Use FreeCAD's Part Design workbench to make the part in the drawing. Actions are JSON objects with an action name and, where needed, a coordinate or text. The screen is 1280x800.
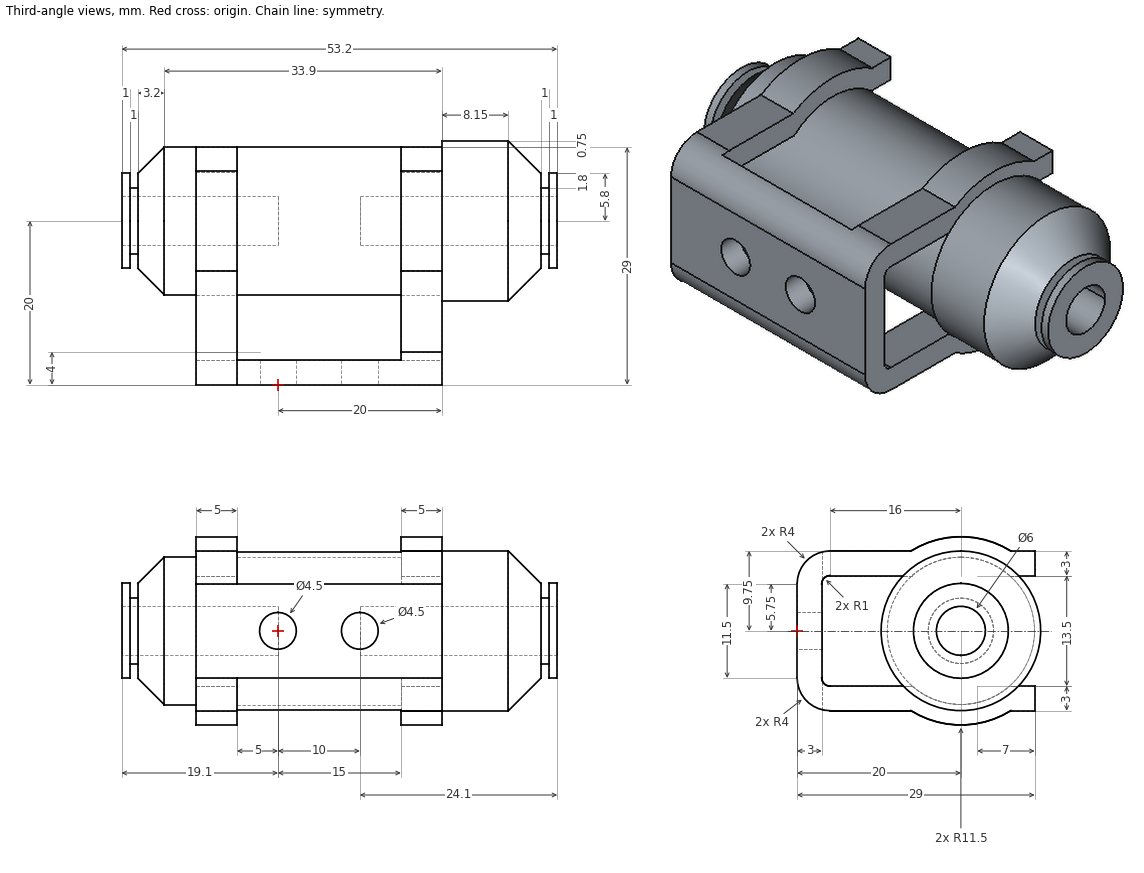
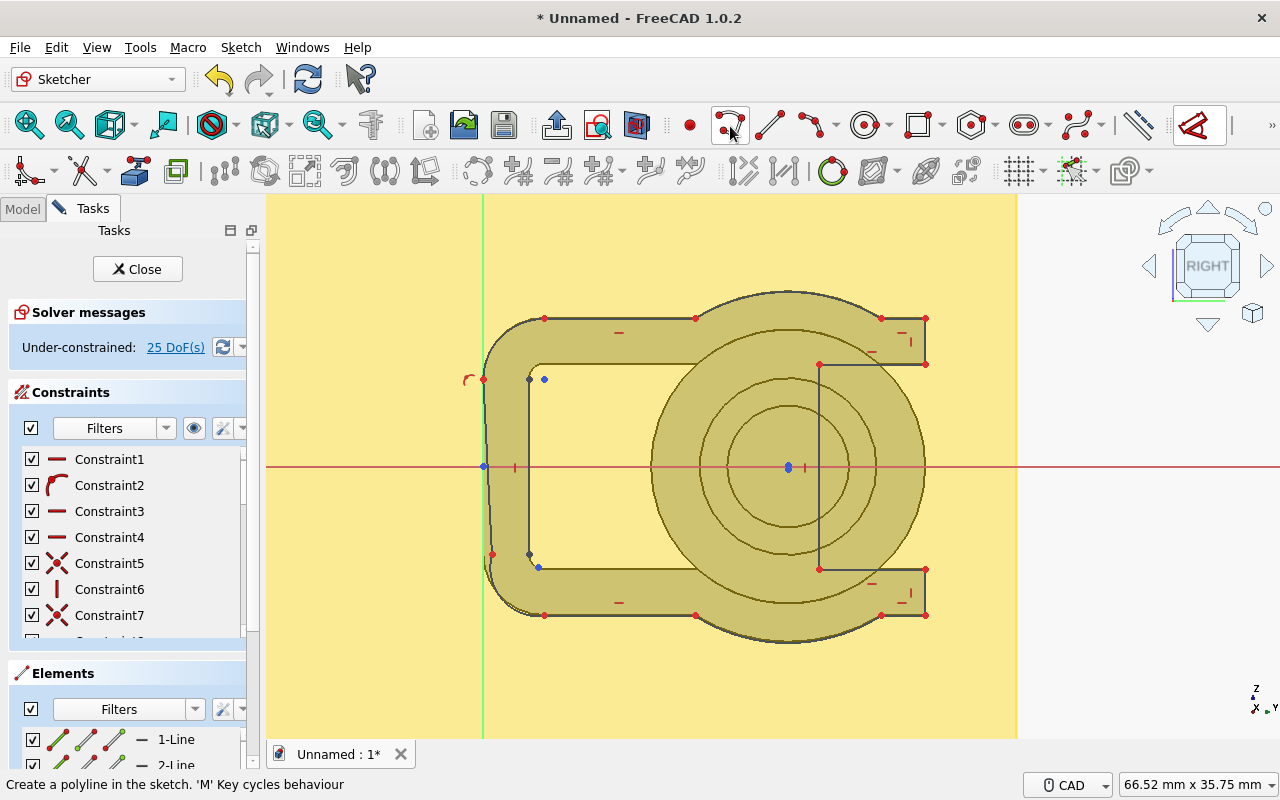
{"action": "left_click", "coordinate": [544, 364]}
{"action": "left_click", "coordinate": [788, 364]}
{"action": "left_click", "coordinate": [788, 569]}
{"action": "left_click", "coordinate": [544, 569]}
{"action": "right_click", "coordinate": [544, 569]}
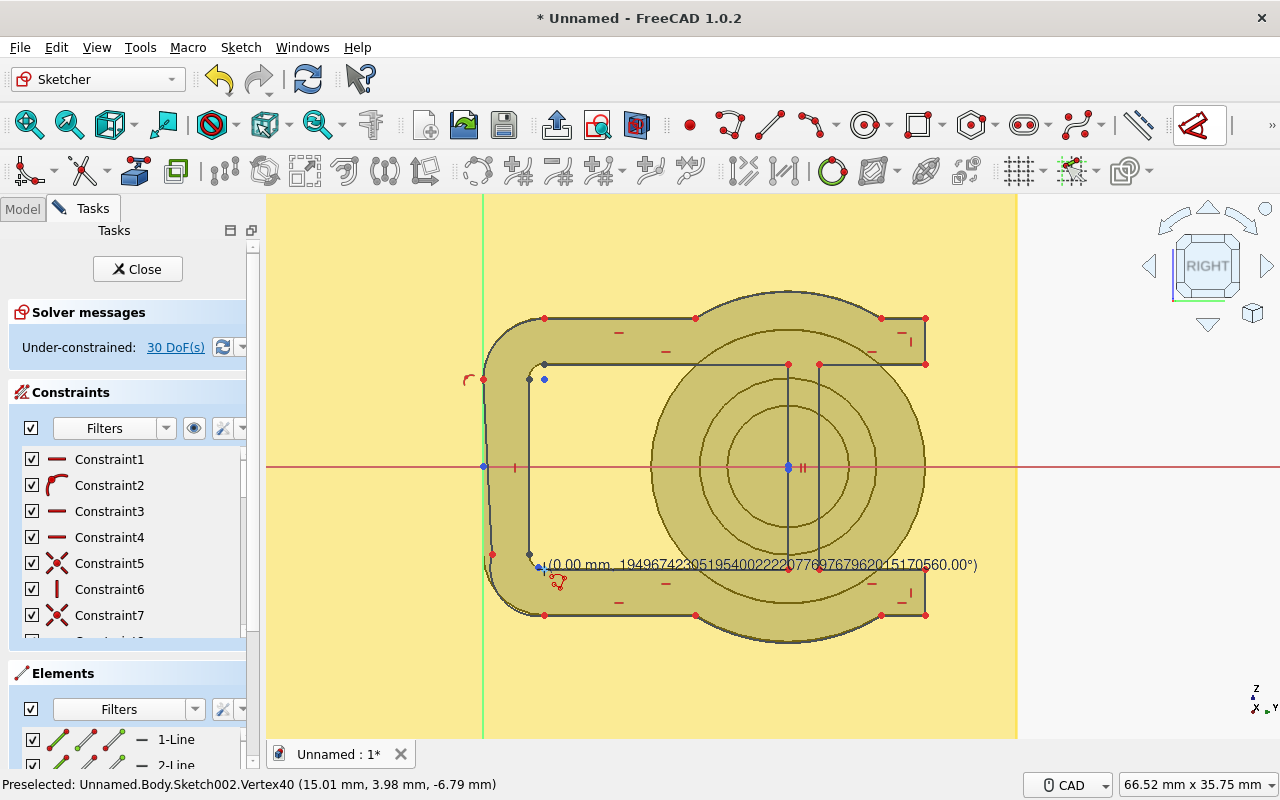
{"action": "left_click", "coordinate": [812, 126]}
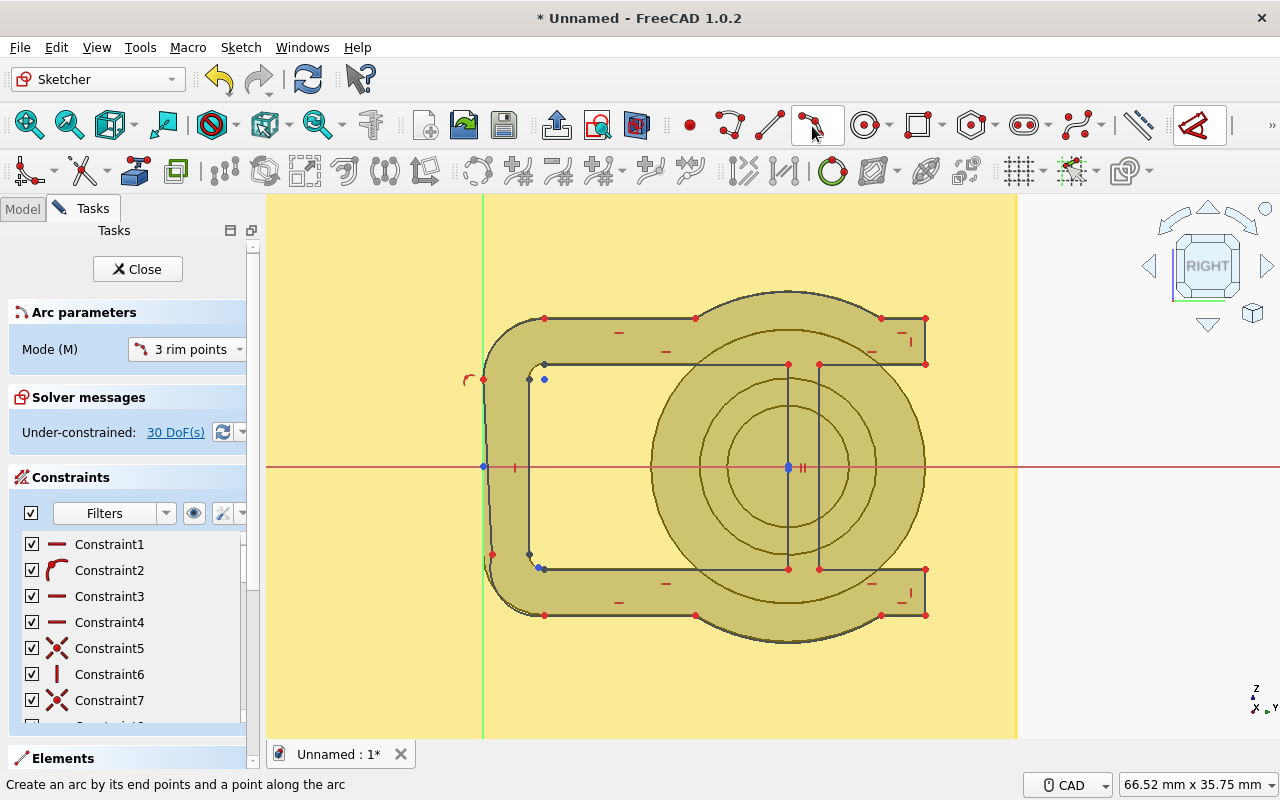
{"action": "left_click", "coordinate": [529, 380]}
{"action": "left_click", "coordinate": [544, 365]}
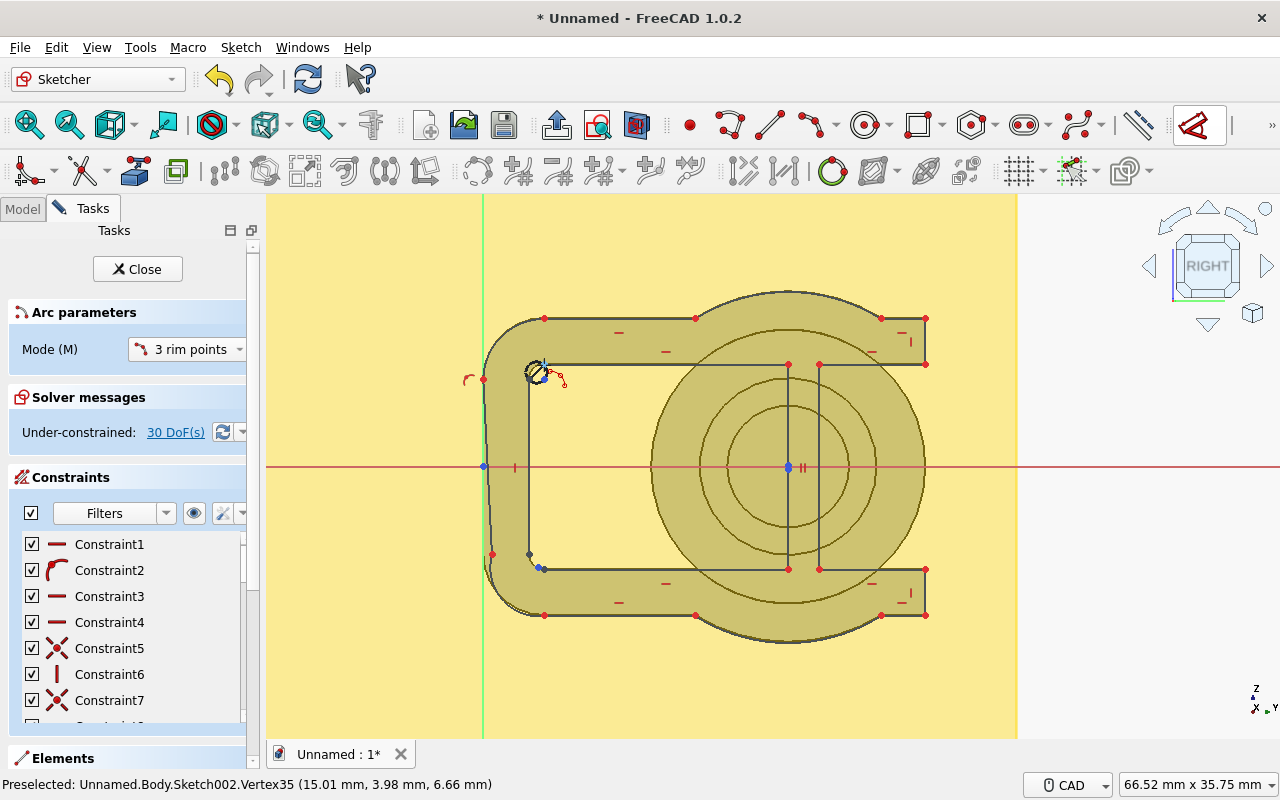
{"action": "scroll", "coordinate": [533, 368], "scroll_direction": "up", "scroll_amount": 7}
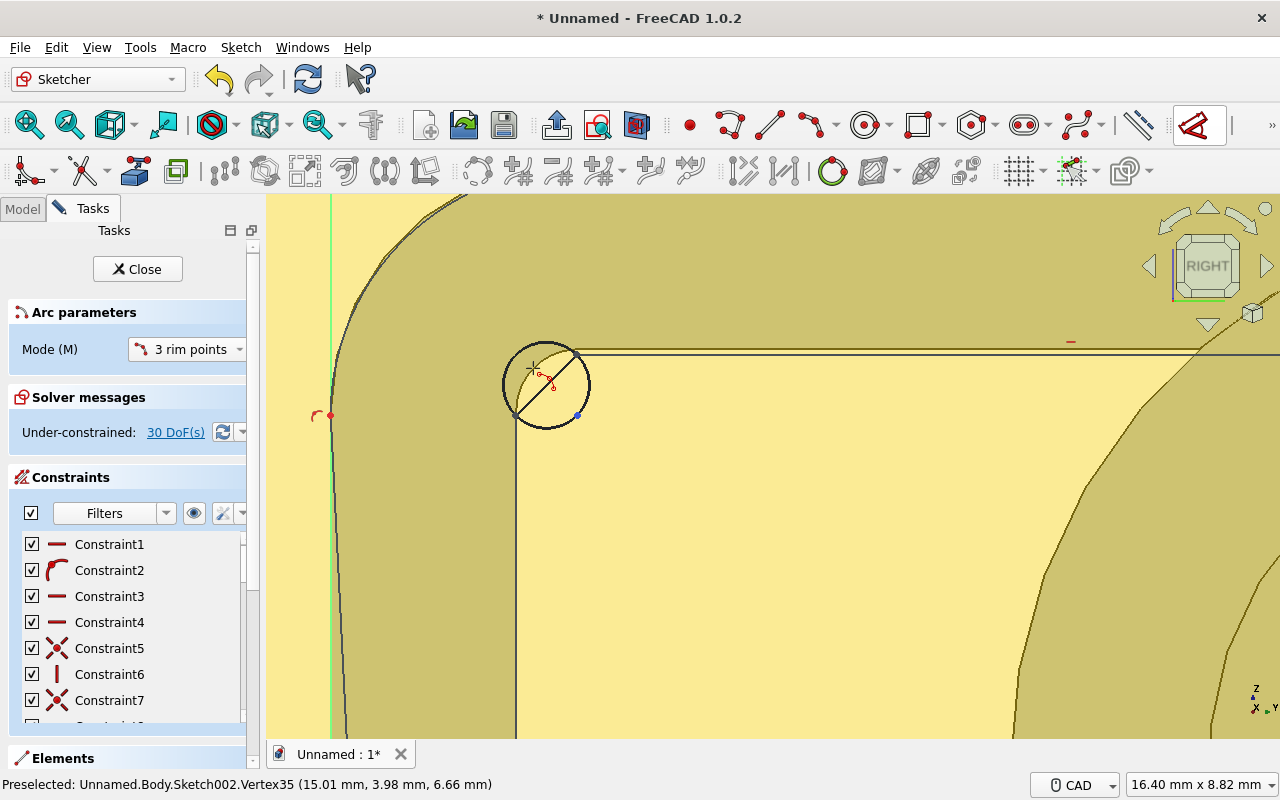
{"action": "left_click", "coordinate": [534, 367]}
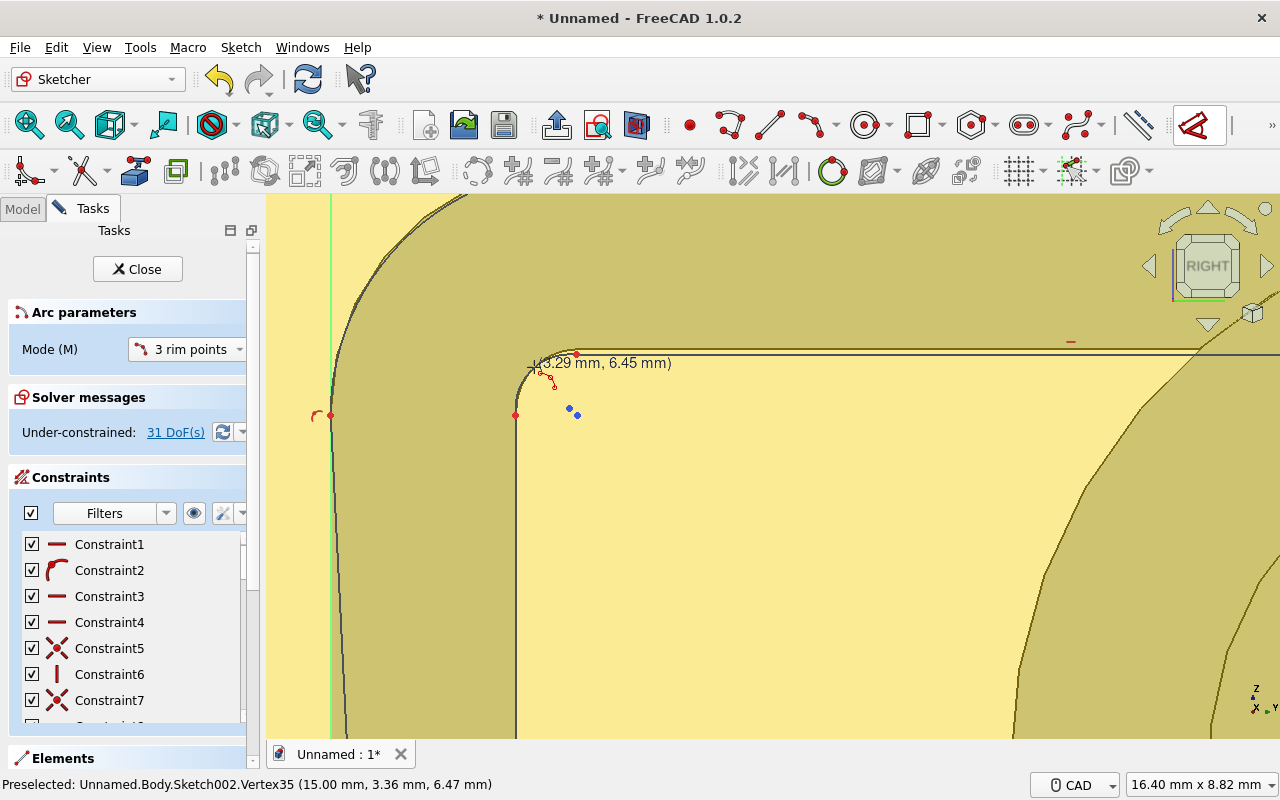
{"action": "scroll", "coordinate": [533, 368], "scroll_direction": "down", "scroll_amount": 7}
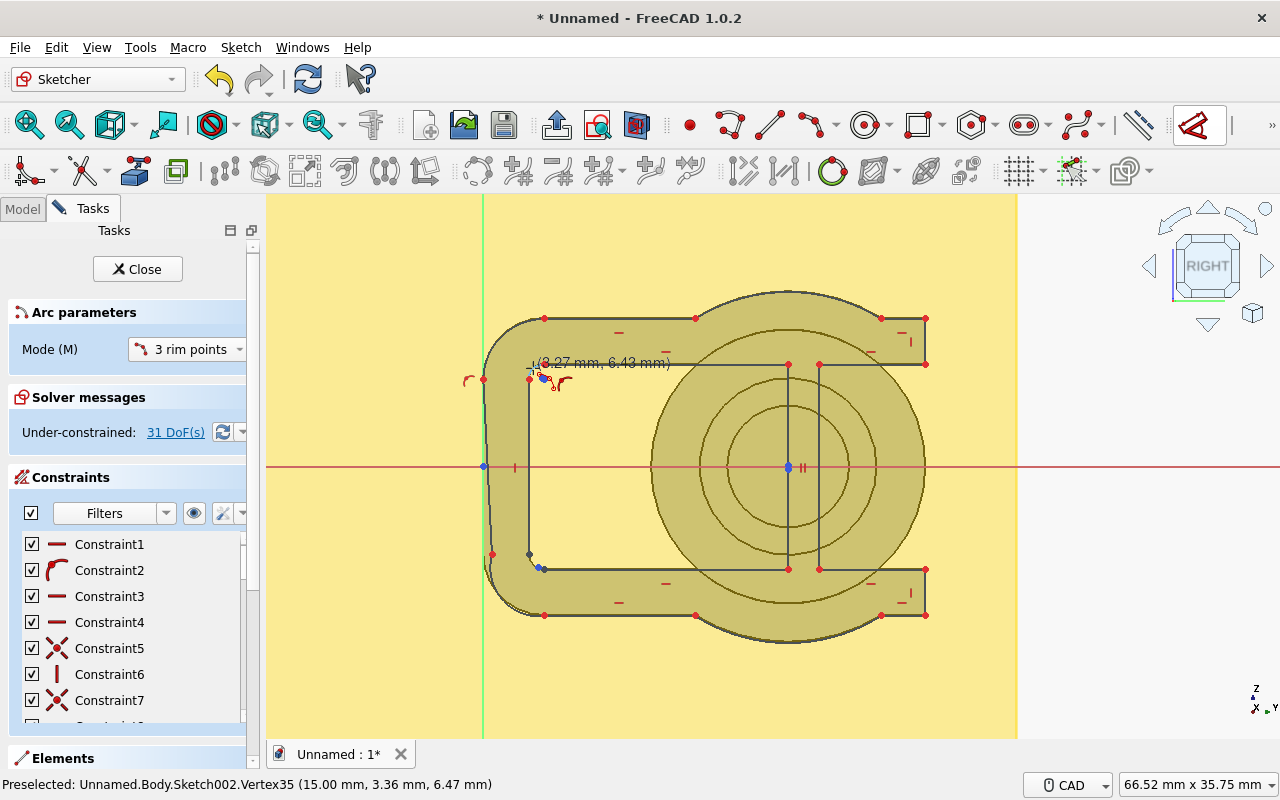
{"action": "left_click", "coordinate": [544, 570]}
{"action": "left_click", "coordinate": [529, 555]}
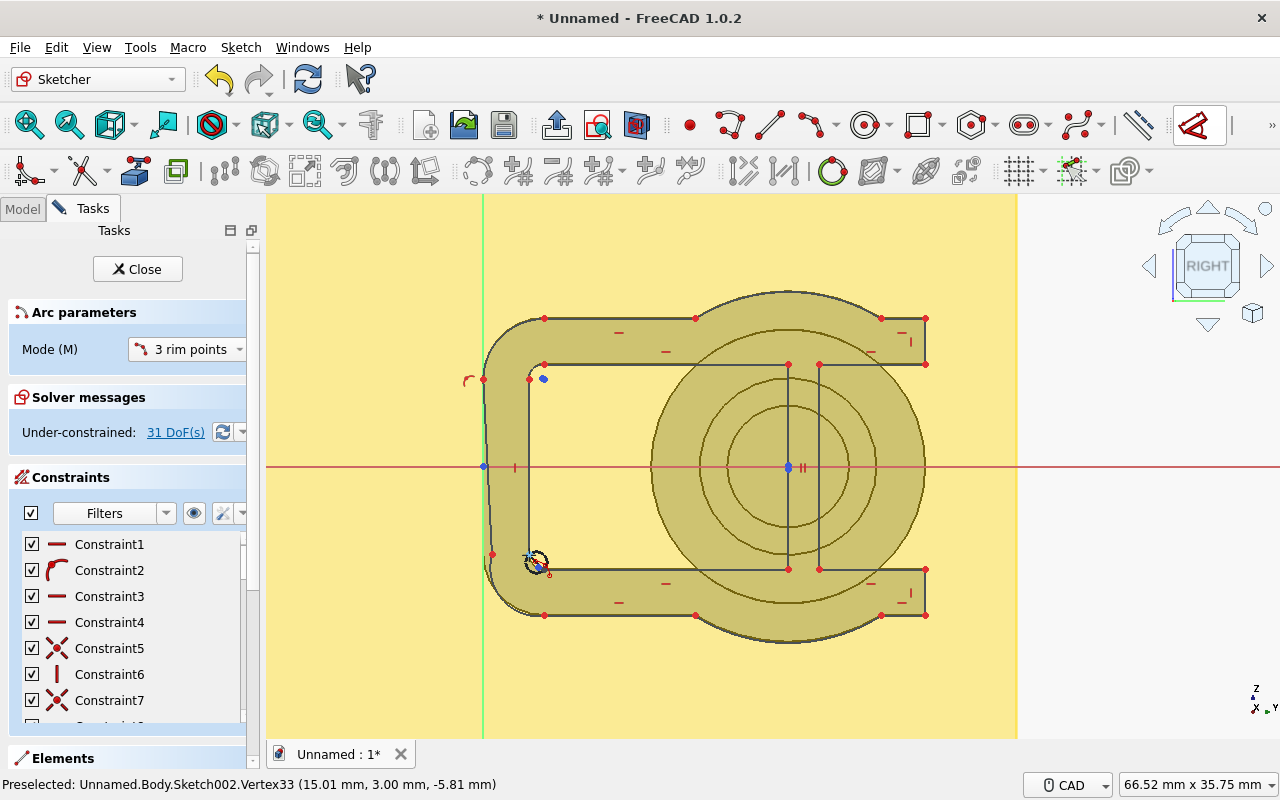
{"action": "scroll", "coordinate": [534, 565], "scroll_direction": "up", "scroll_amount": 7}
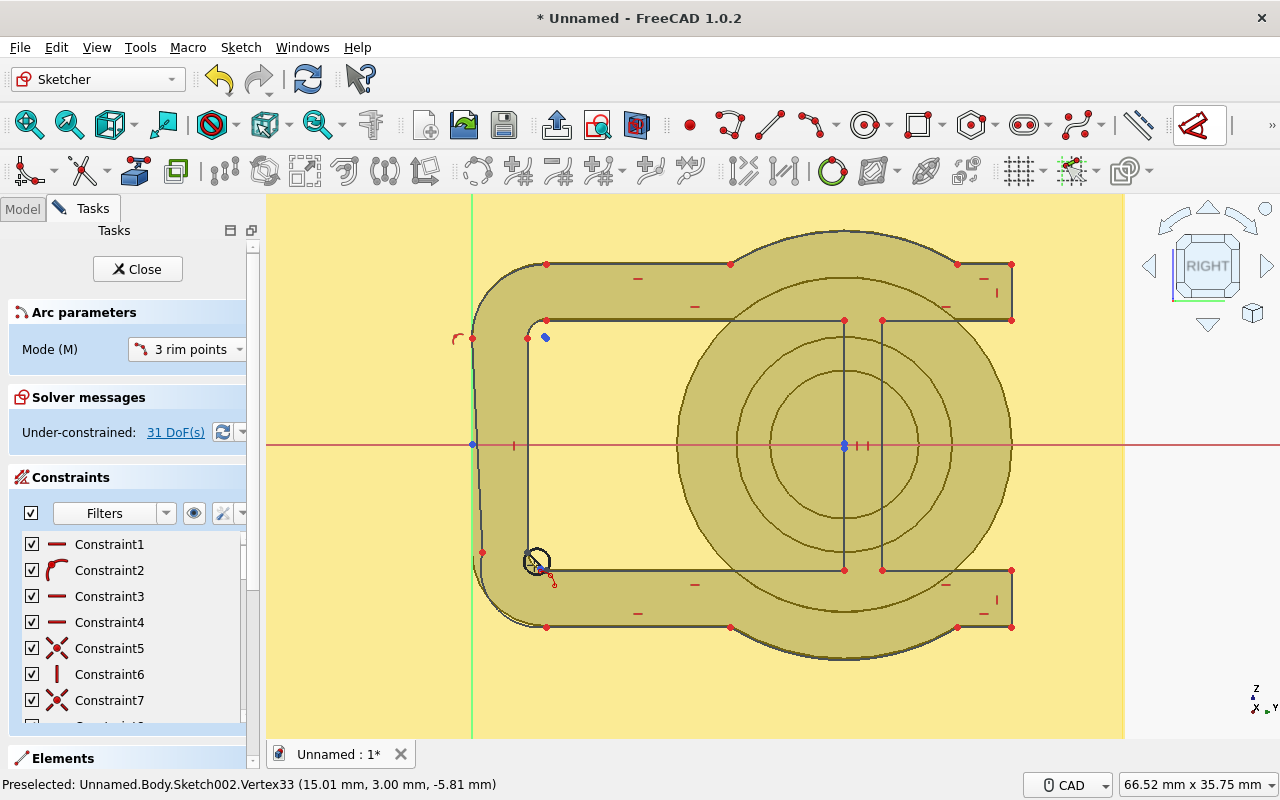
{"action": "left_click", "coordinate": [531, 563]}
{"action": "key", "text": "Escape"}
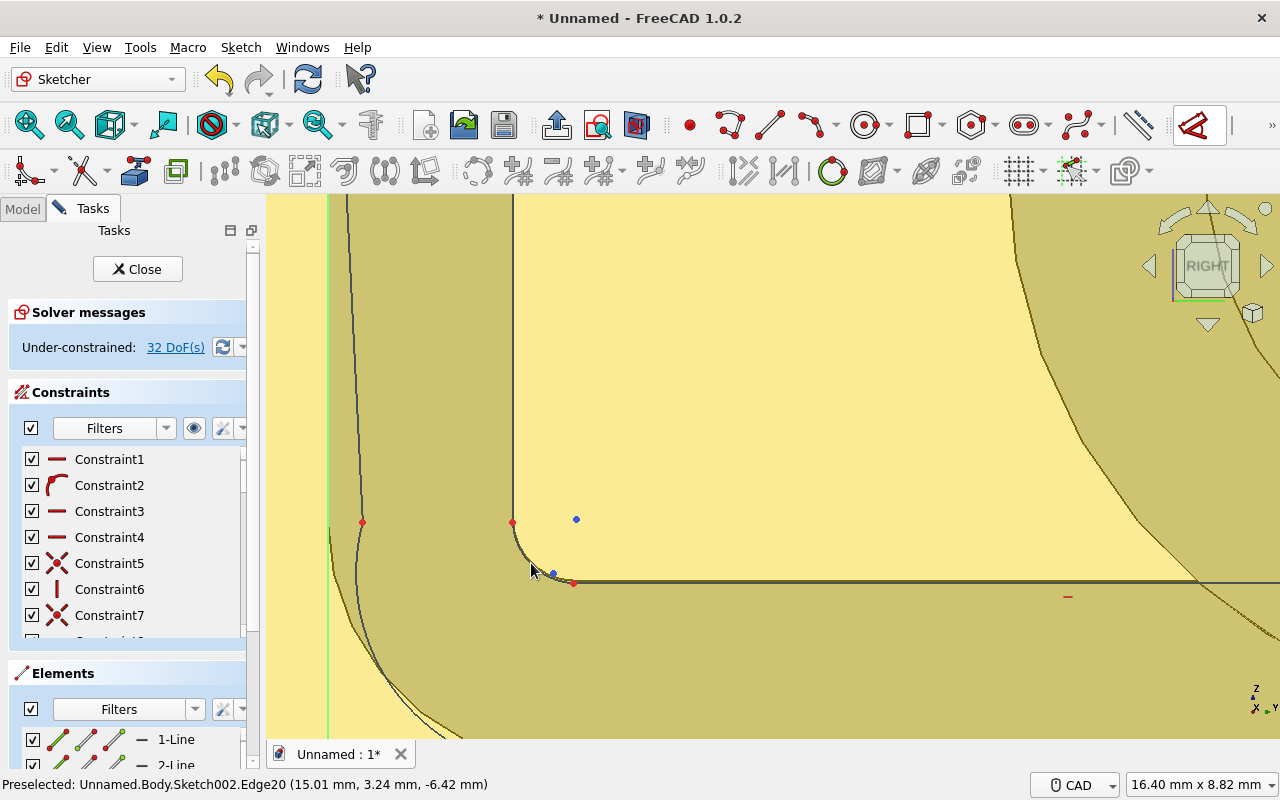
{"action": "scroll", "coordinate": [534, 566], "scroll_direction": "down", "scroll_amount": 7}